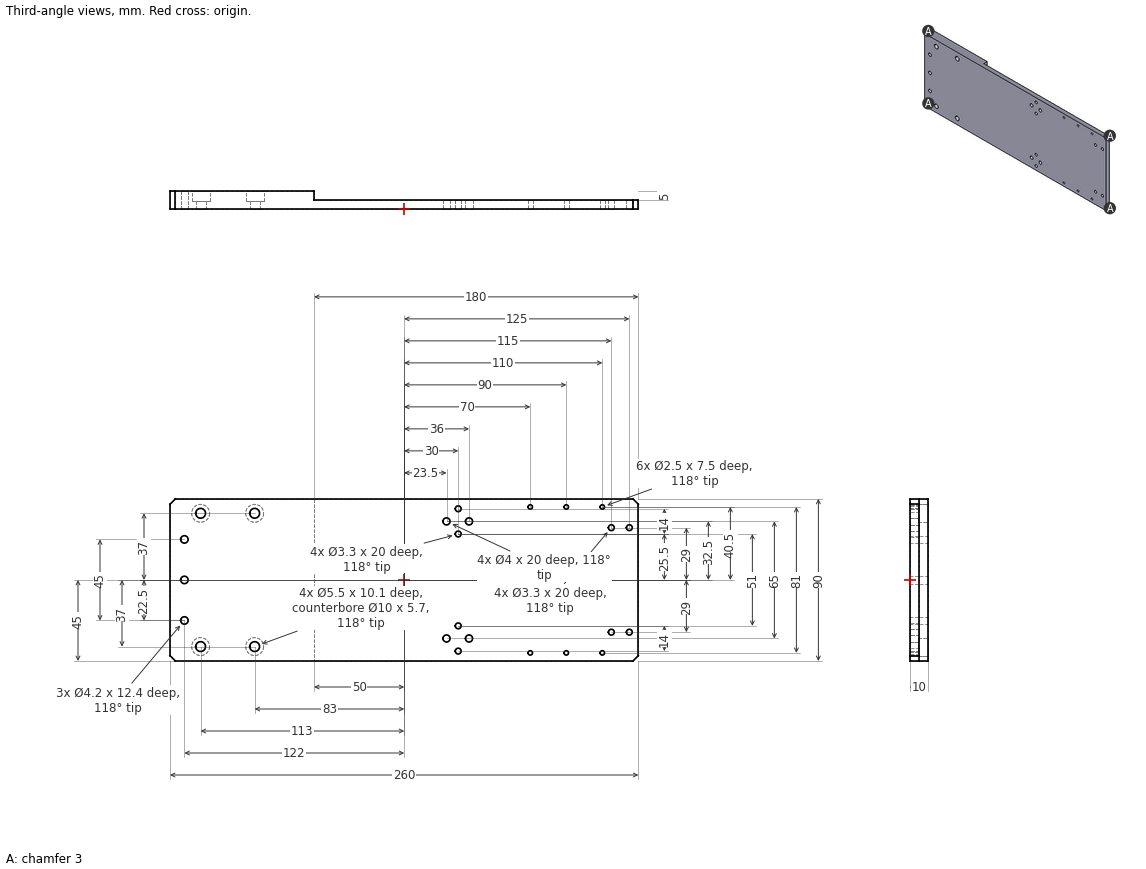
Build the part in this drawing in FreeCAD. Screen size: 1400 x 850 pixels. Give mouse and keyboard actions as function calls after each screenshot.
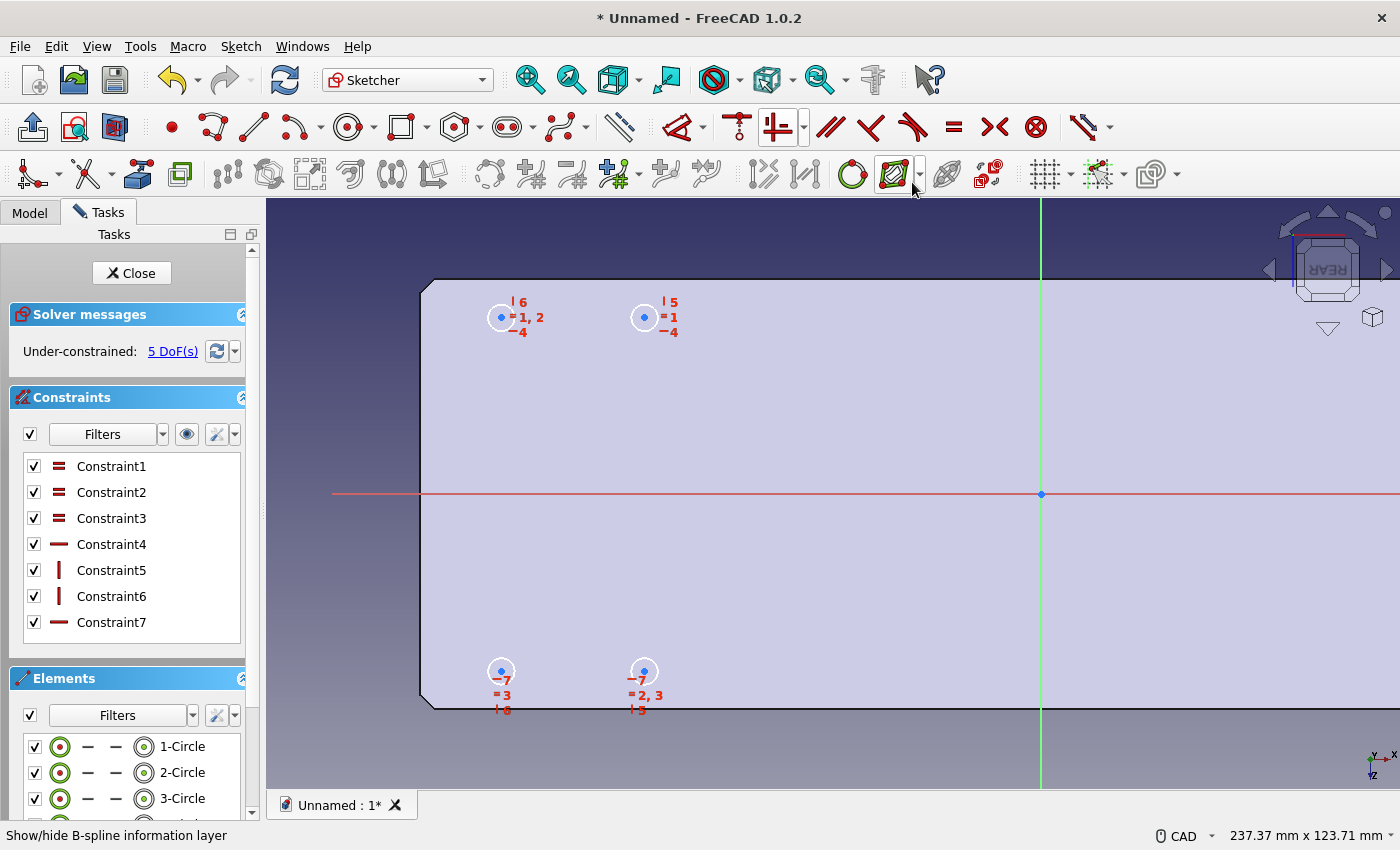
click(676, 128)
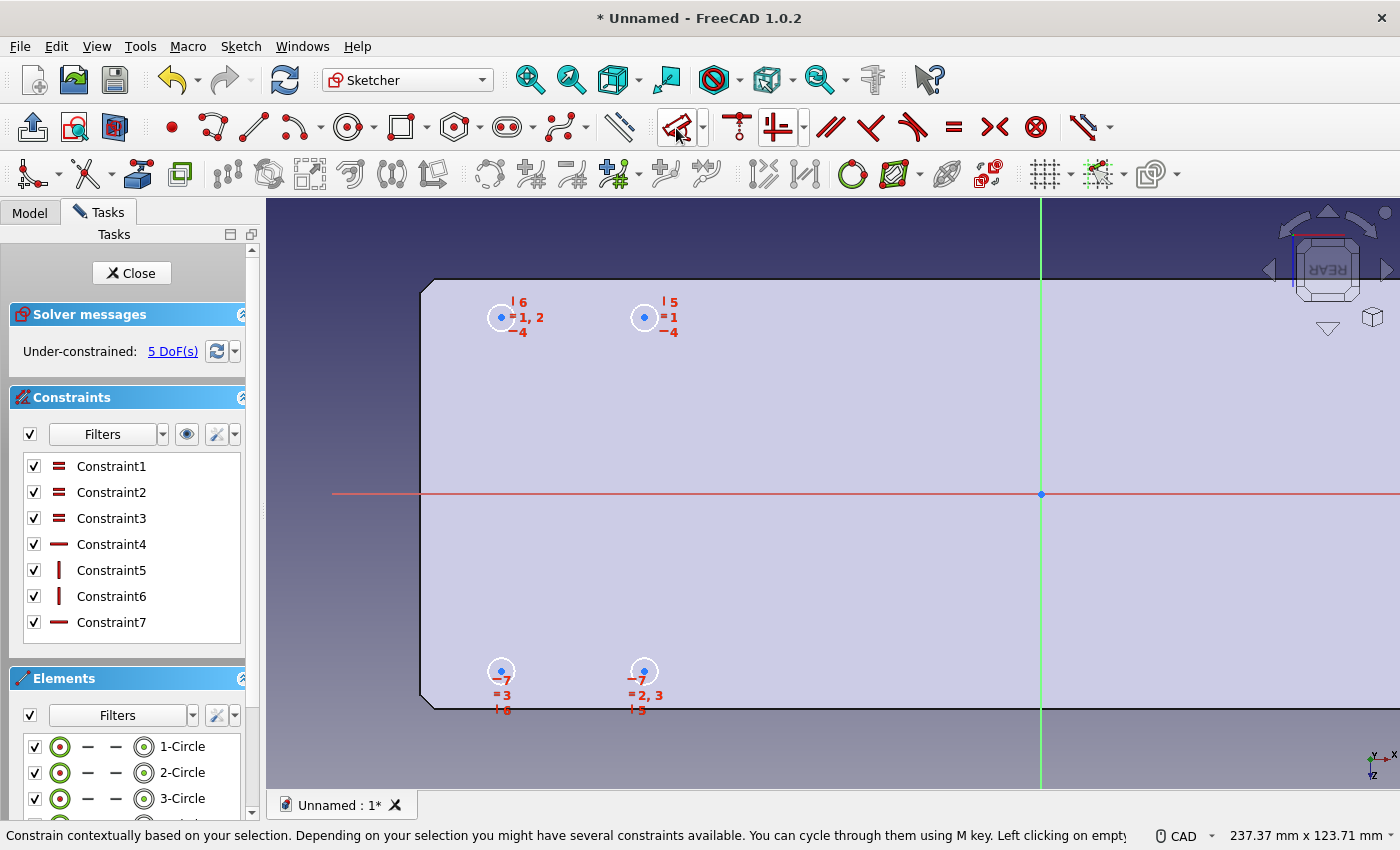
scroll(654, 309, up, 3)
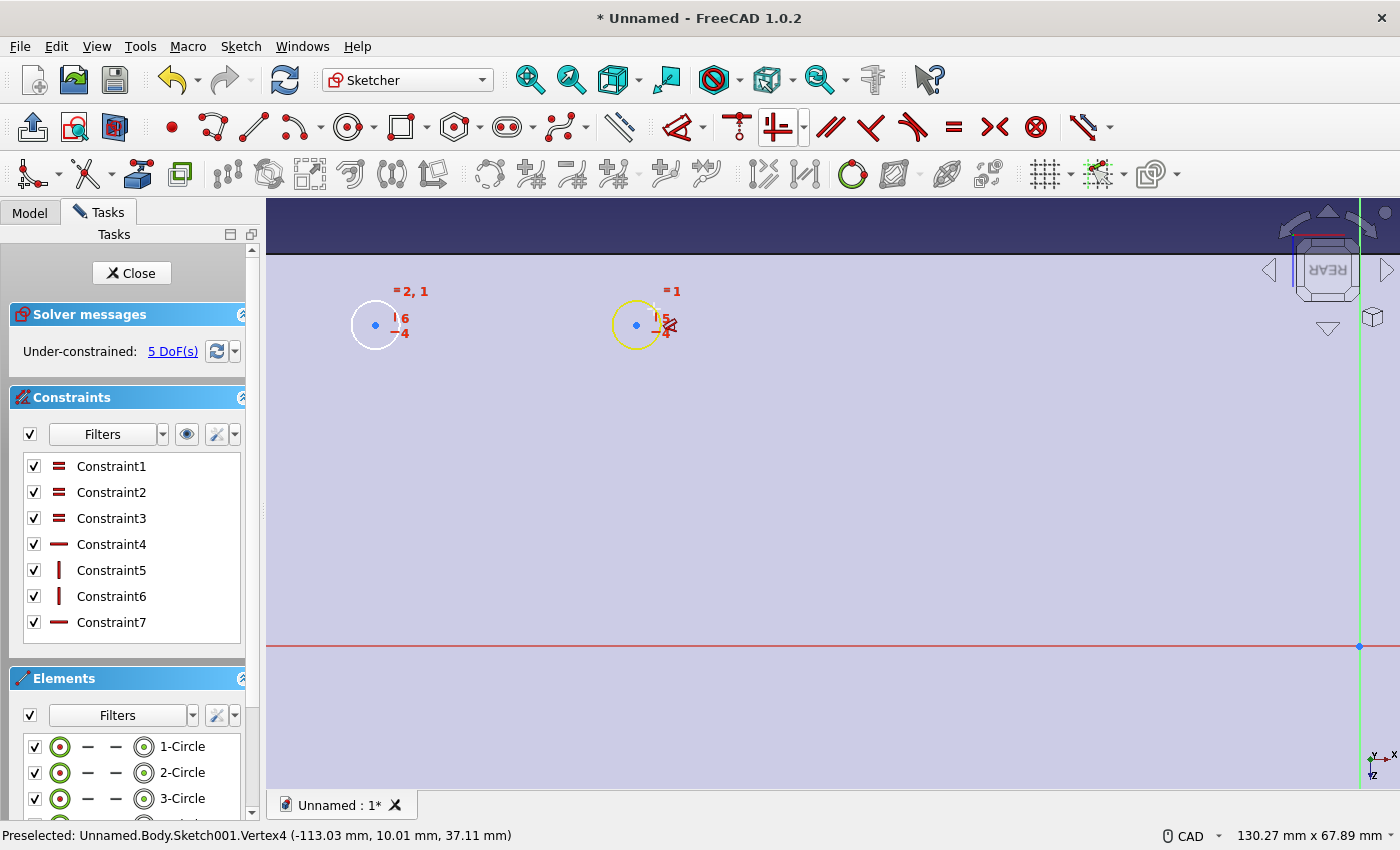
click(654, 308)
click(677, 286)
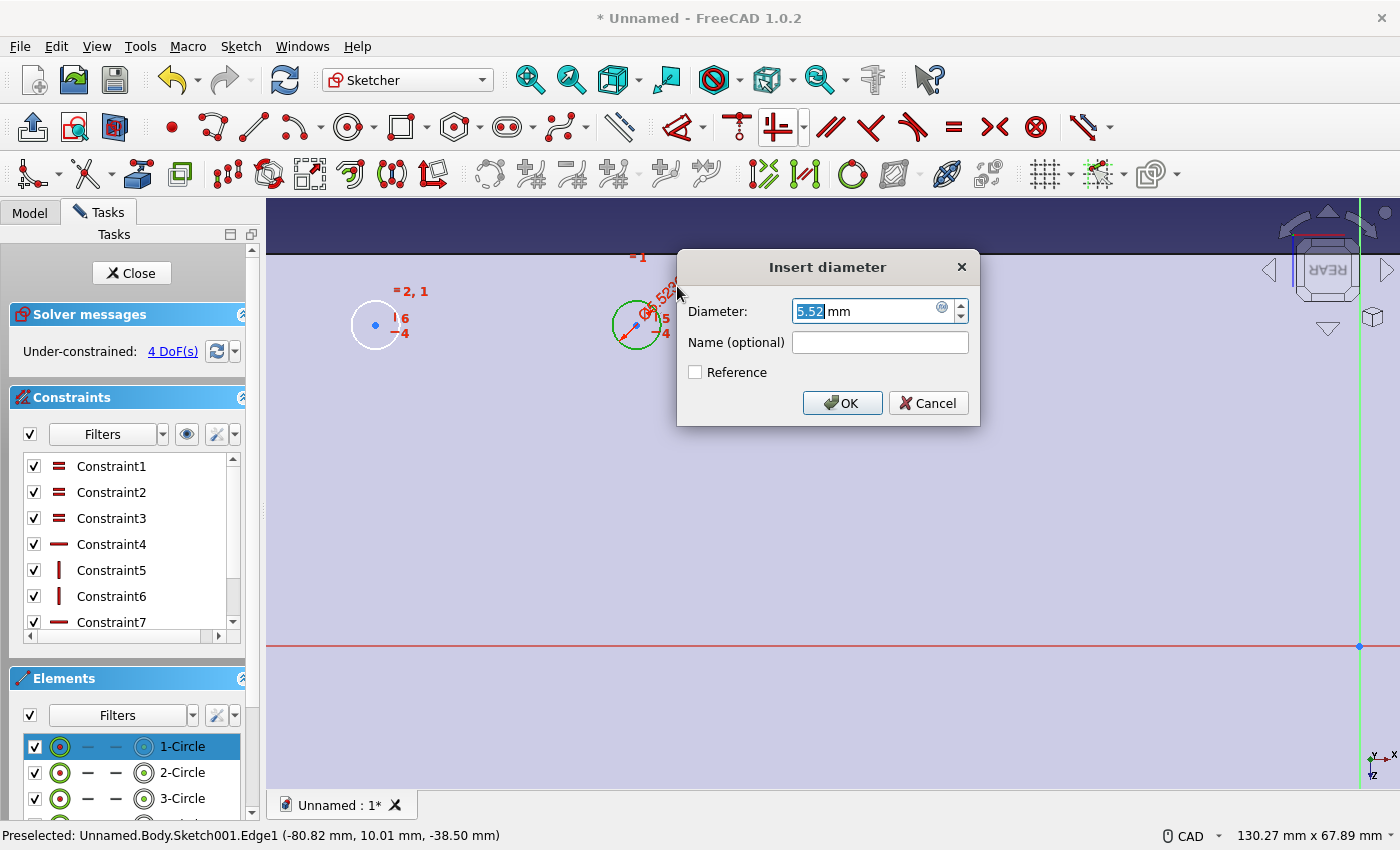
text(5.5)
key(Return)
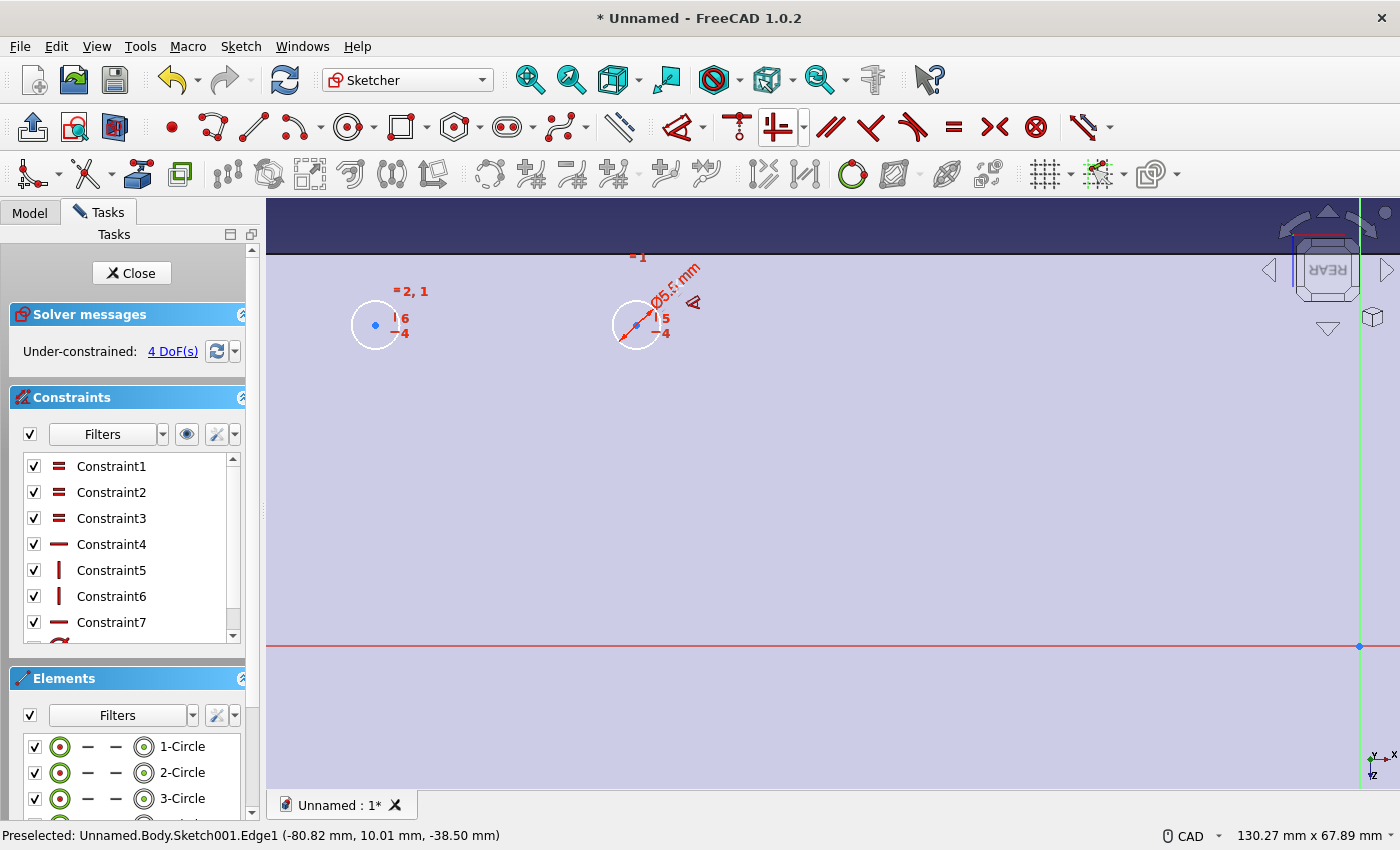
click(637, 325)
click(936, 291)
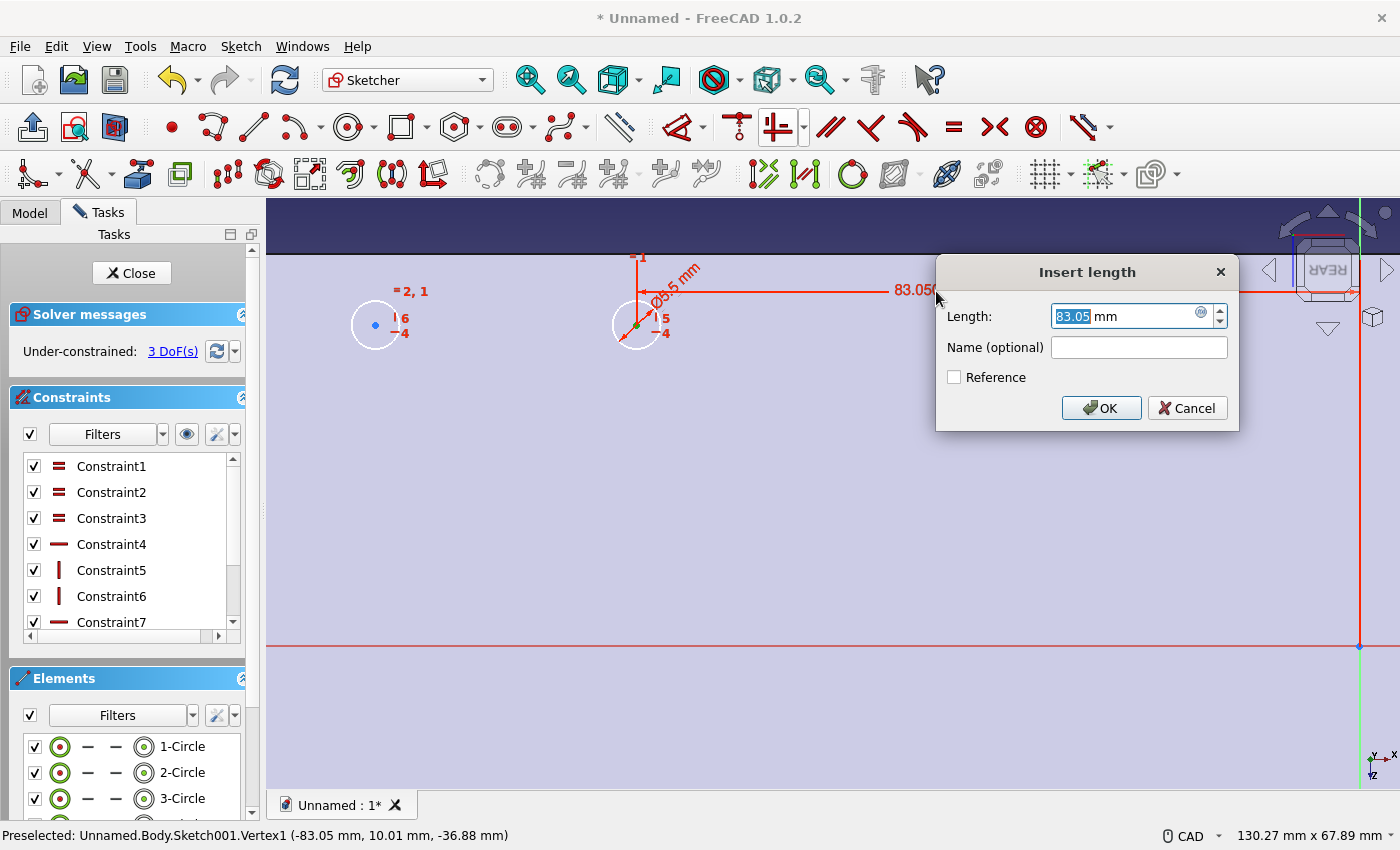
text(83)
key(Return)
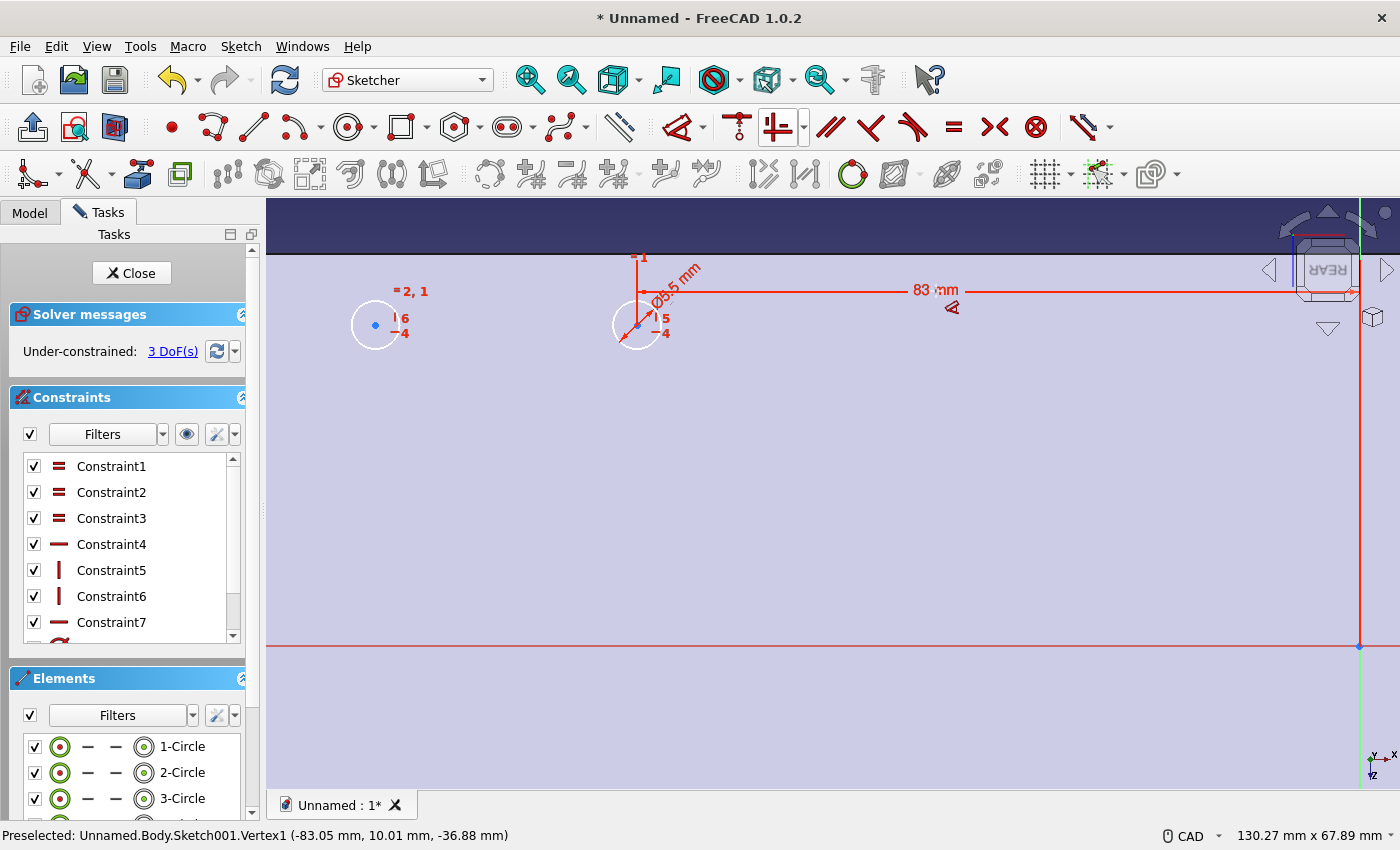
click(637, 325)
click(603, 486)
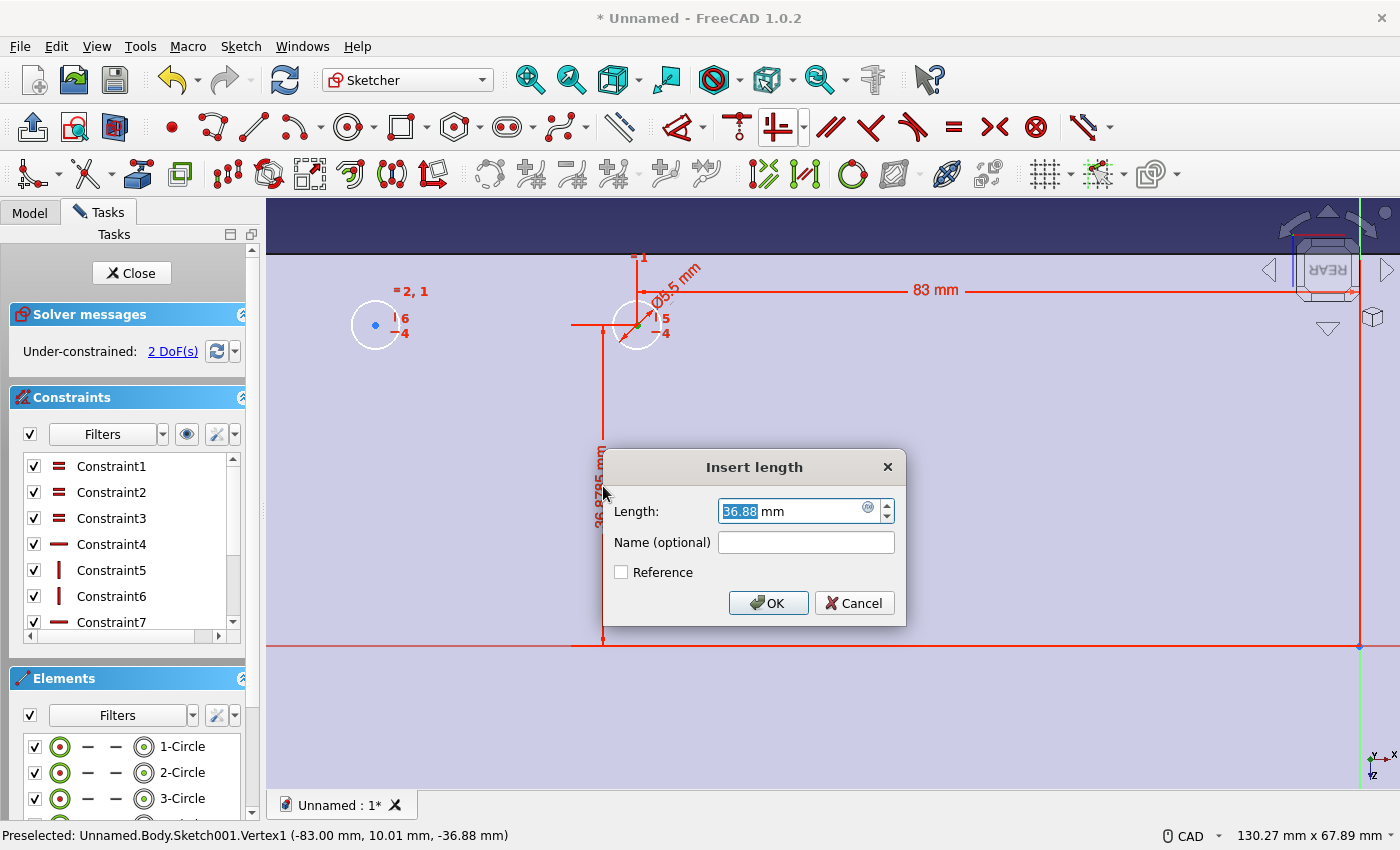
text(37)
key(Return)